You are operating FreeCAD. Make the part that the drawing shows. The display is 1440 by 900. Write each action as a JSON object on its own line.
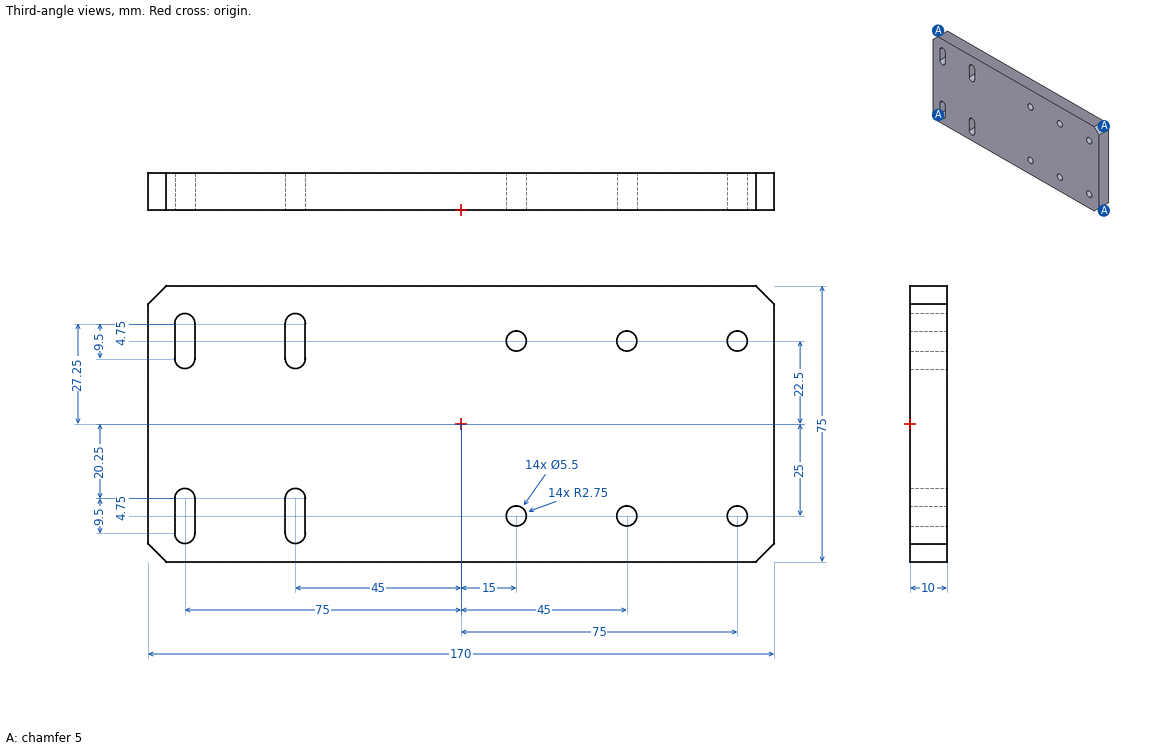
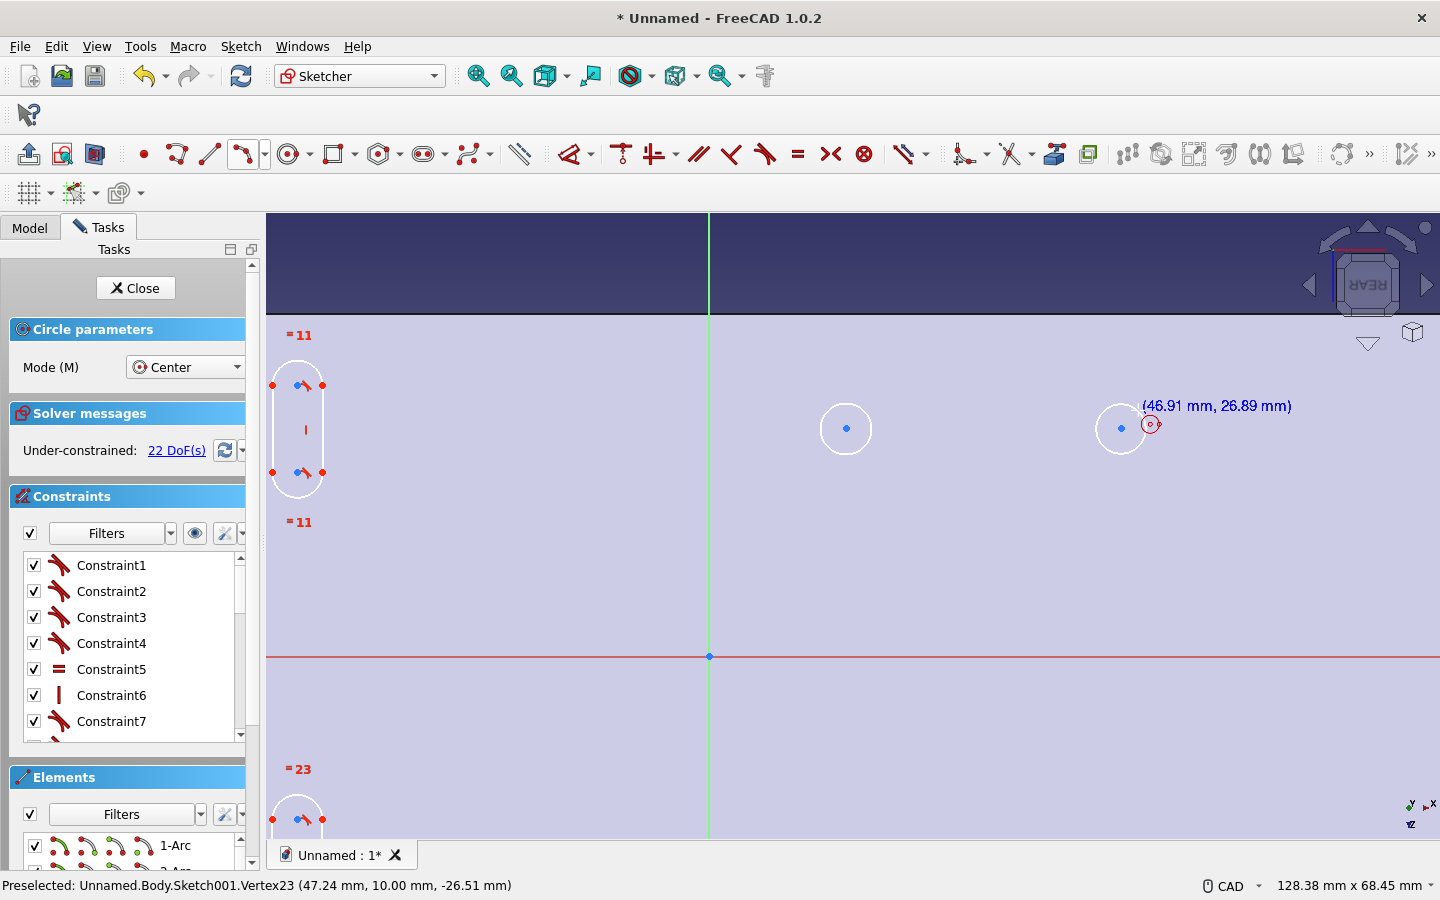
{"action": "scroll", "coordinate": [846, 429], "scroll_direction": "down", "scroll_amount": 4}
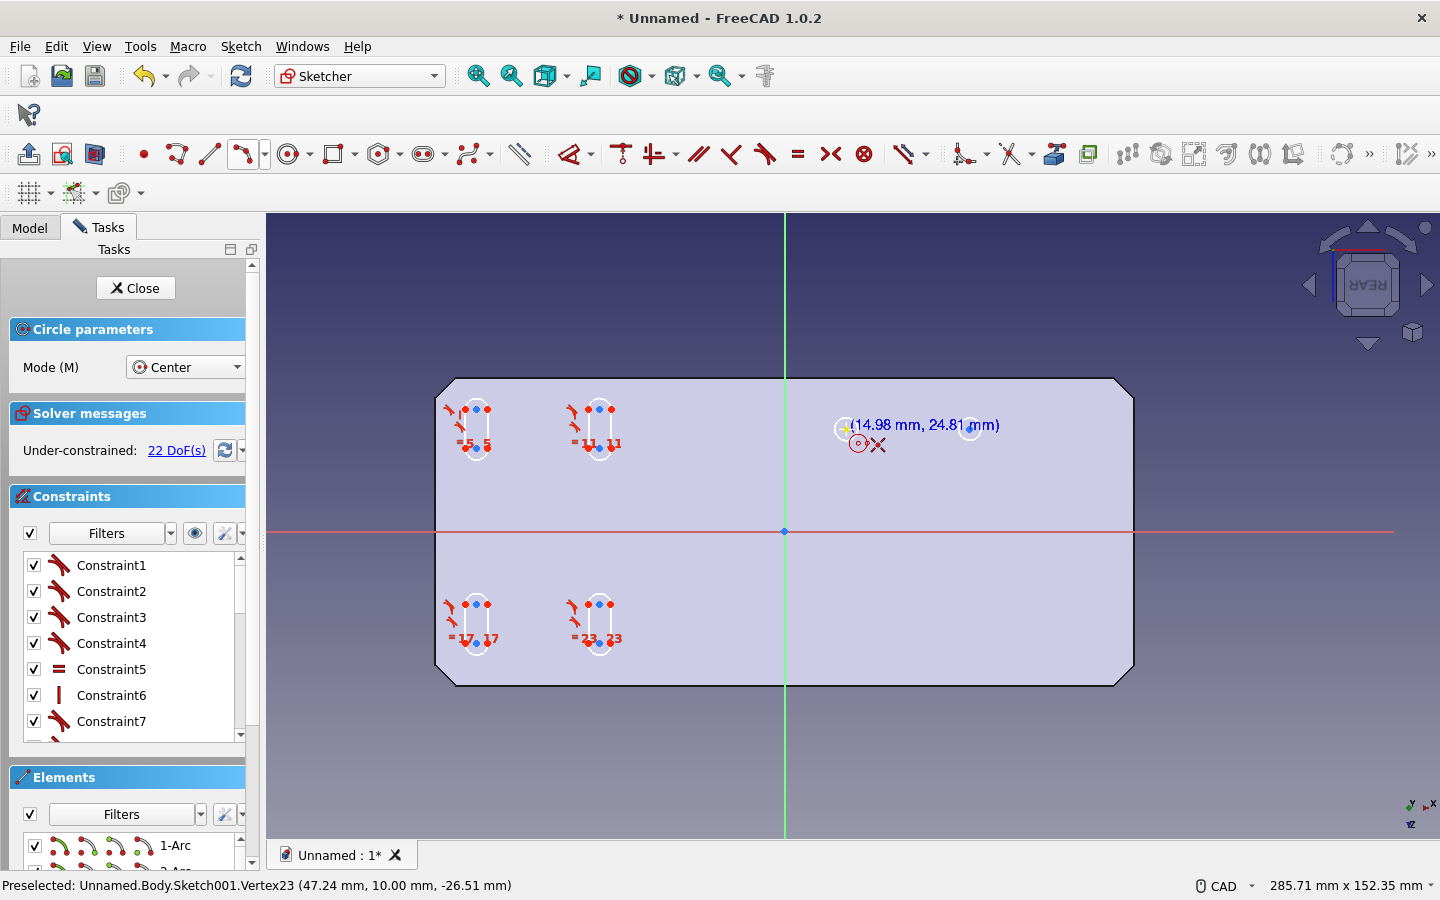
{"action": "scroll", "coordinate": [1093, 429], "scroll_direction": "up", "scroll_amount": 4}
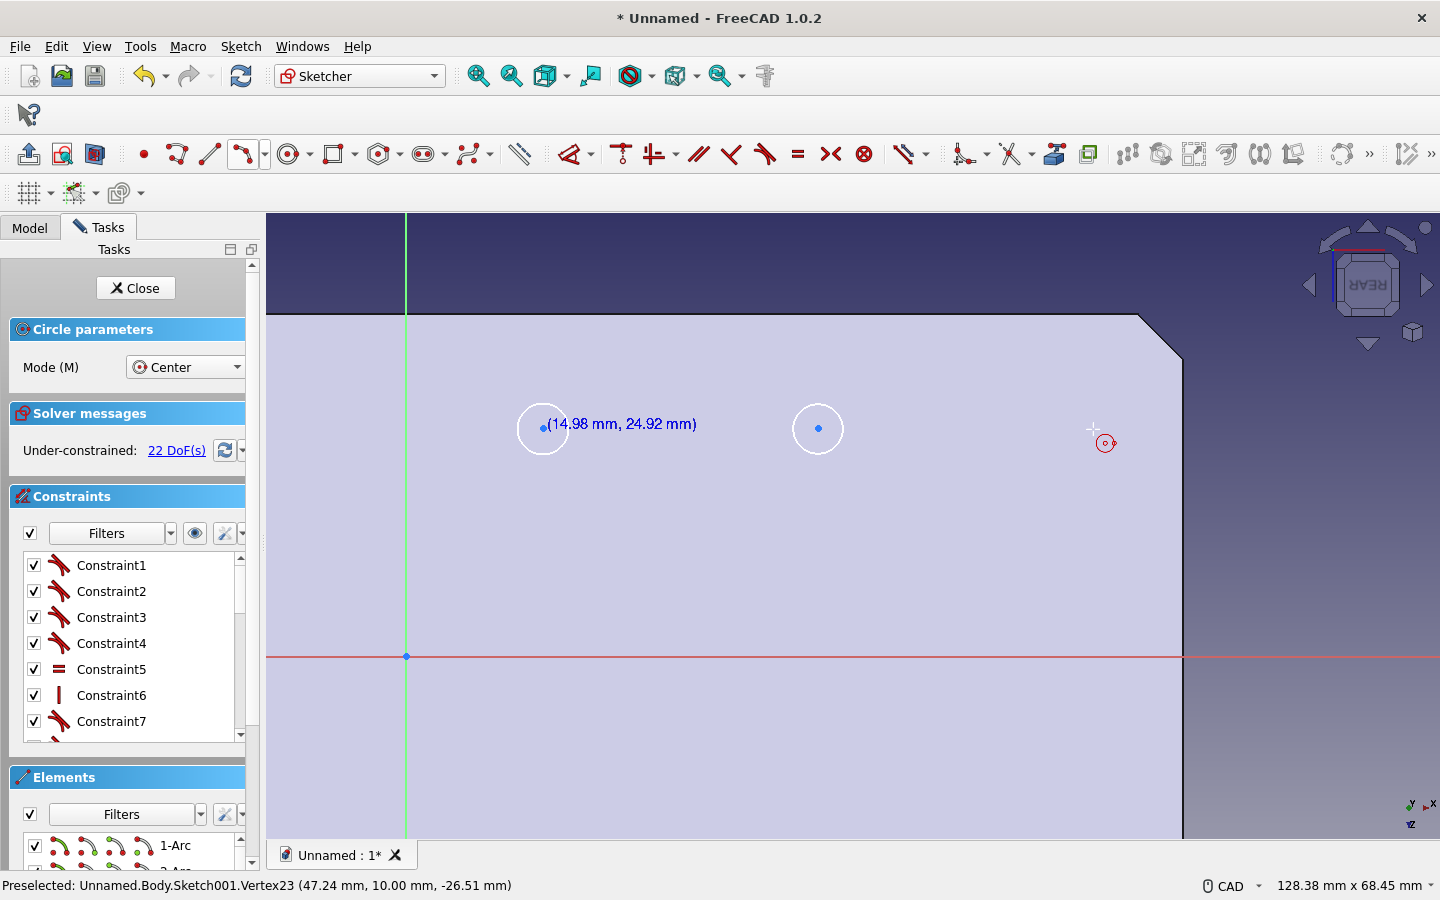
{"action": "left_click", "coordinate": [1092, 428]}
{"action": "left_click", "coordinate": [1110, 410]}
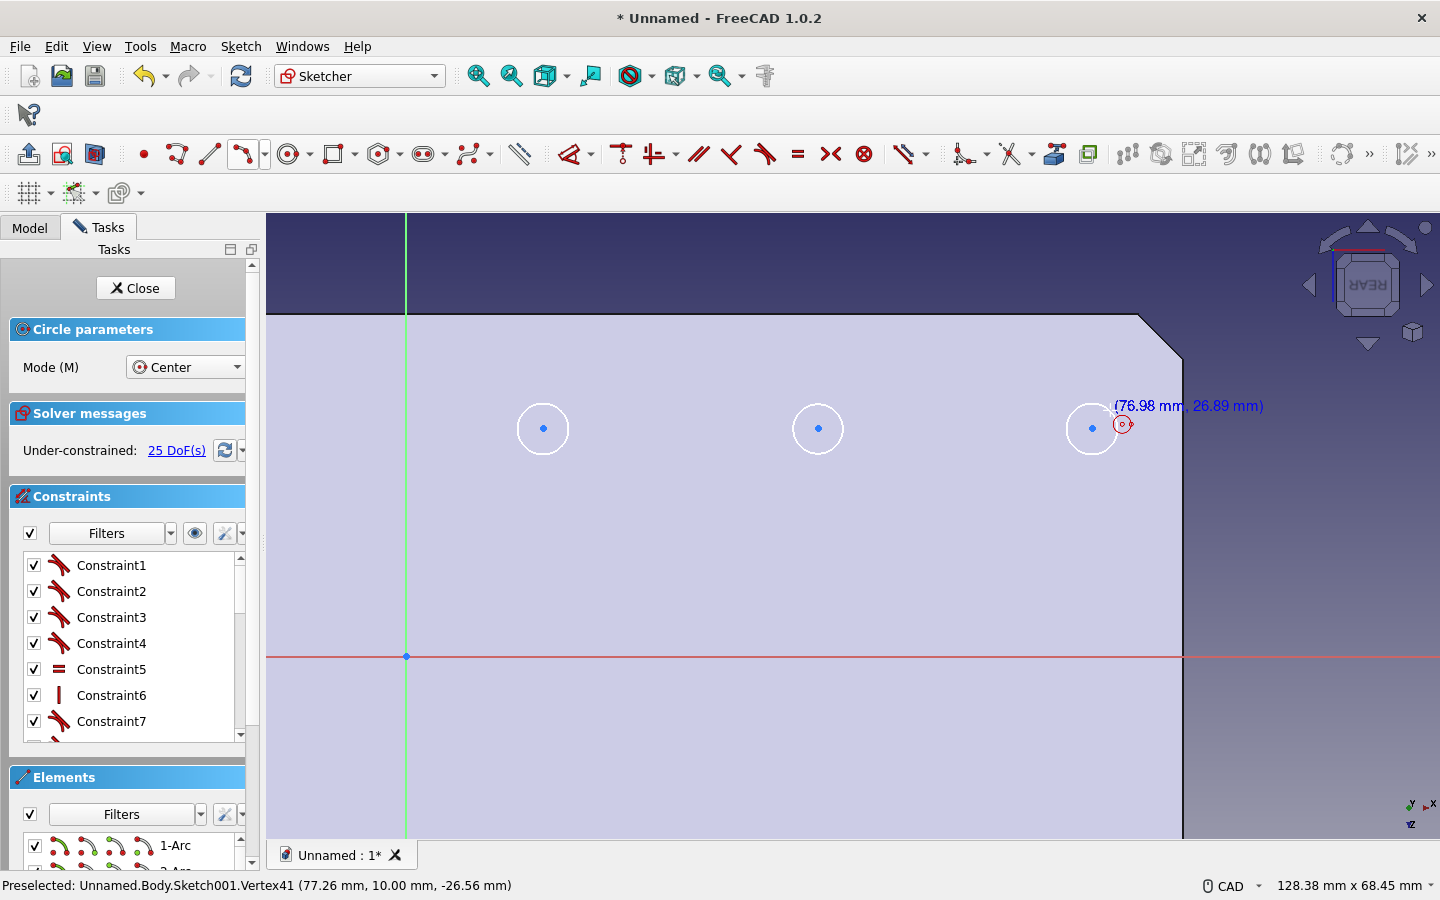
{"action": "scroll", "coordinate": [1093, 429], "scroll_direction": "down", "scroll_amount": 4}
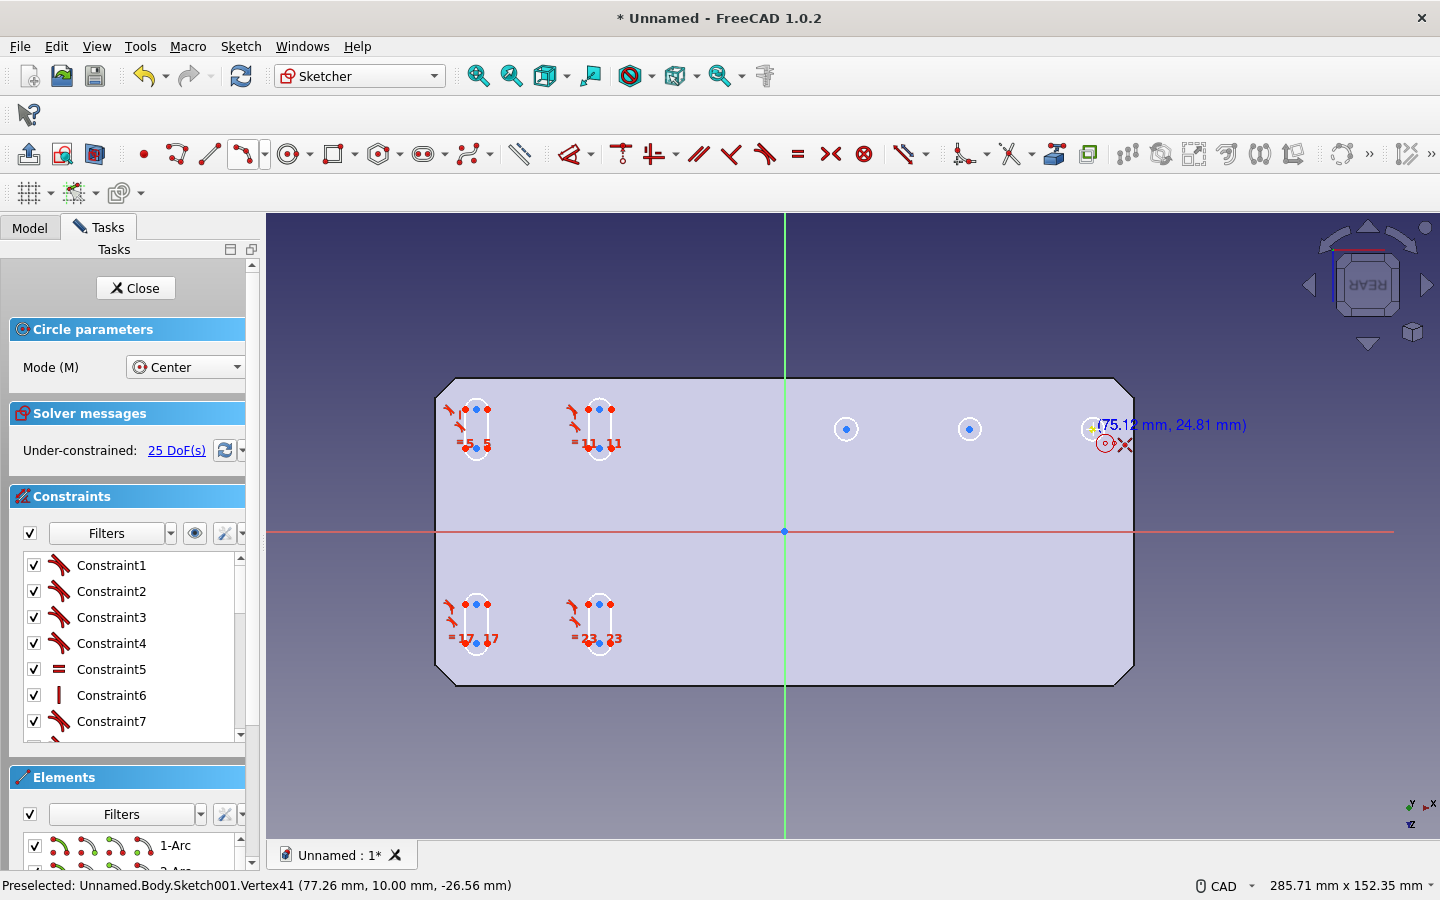
{"action": "scroll", "coordinate": [846, 624], "scroll_direction": "up", "scroll_amount": 4}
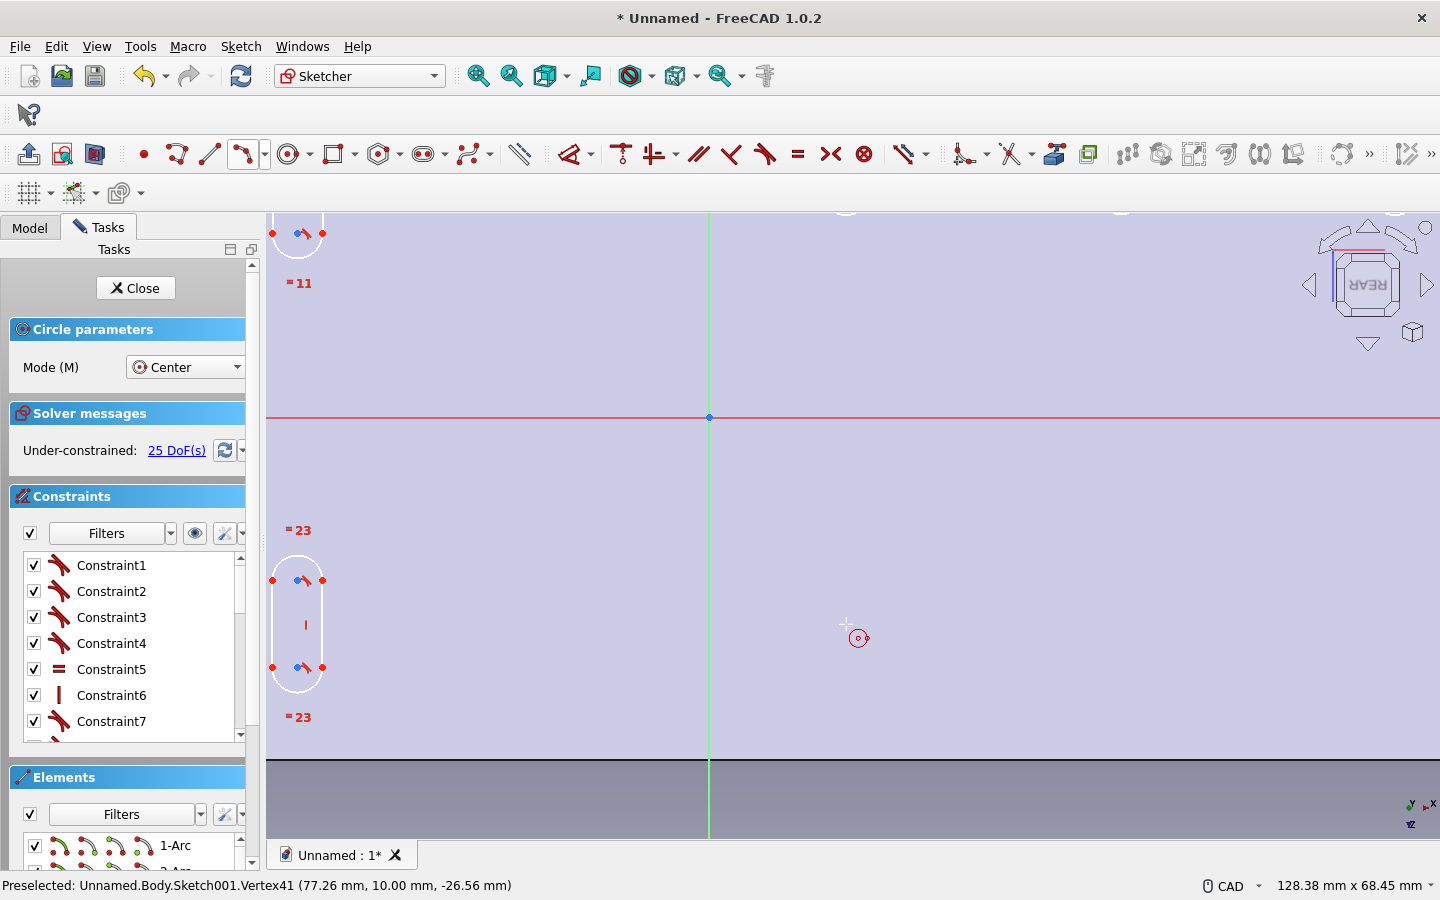
{"action": "left_click", "coordinate": [846, 623]}
{"action": "left_click", "coordinate": [864, 606]}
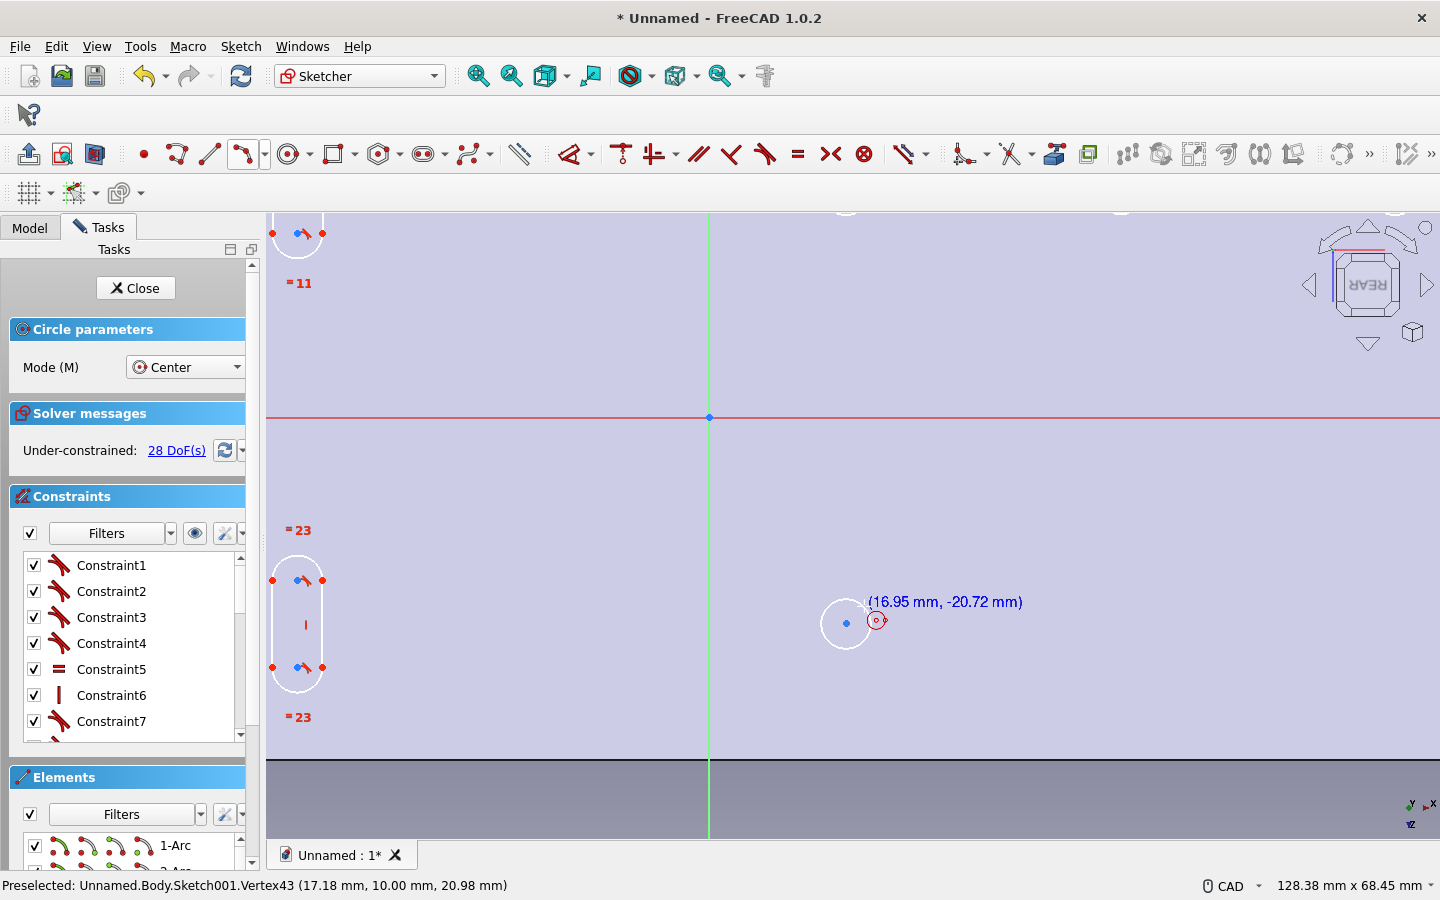
{"action": "left_click", "coordinate": [1121, 623]}
{"action": "left_click", "coordinate": [1138, 606]}